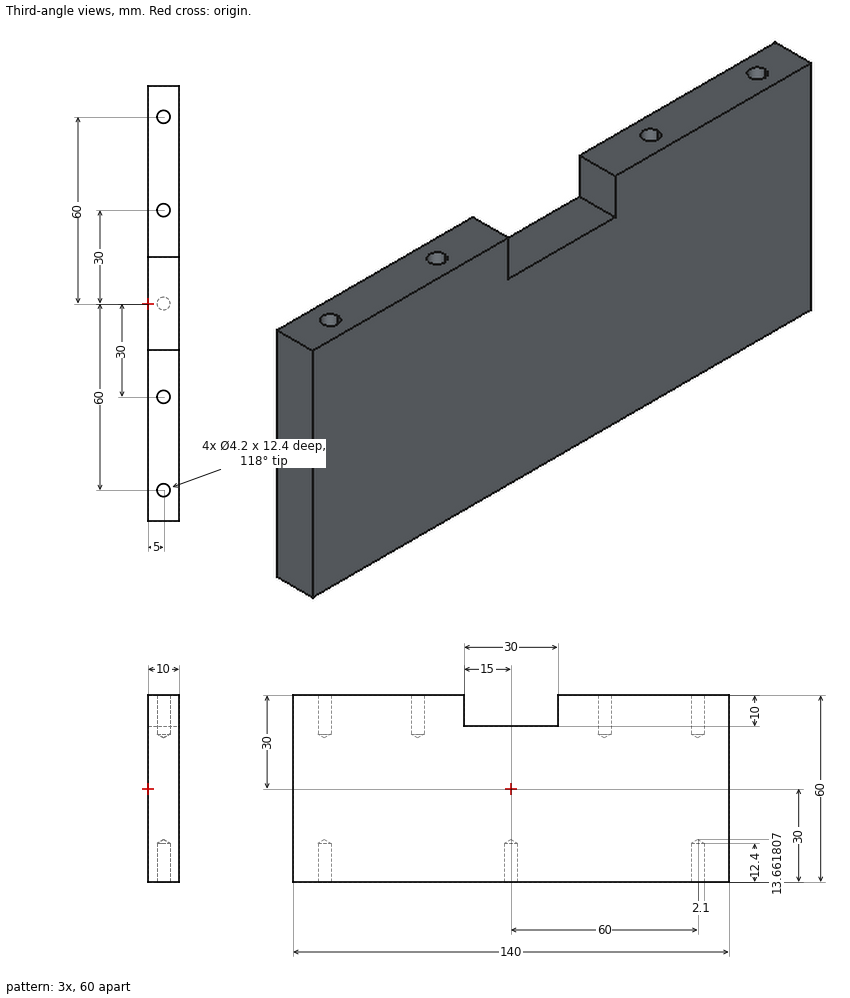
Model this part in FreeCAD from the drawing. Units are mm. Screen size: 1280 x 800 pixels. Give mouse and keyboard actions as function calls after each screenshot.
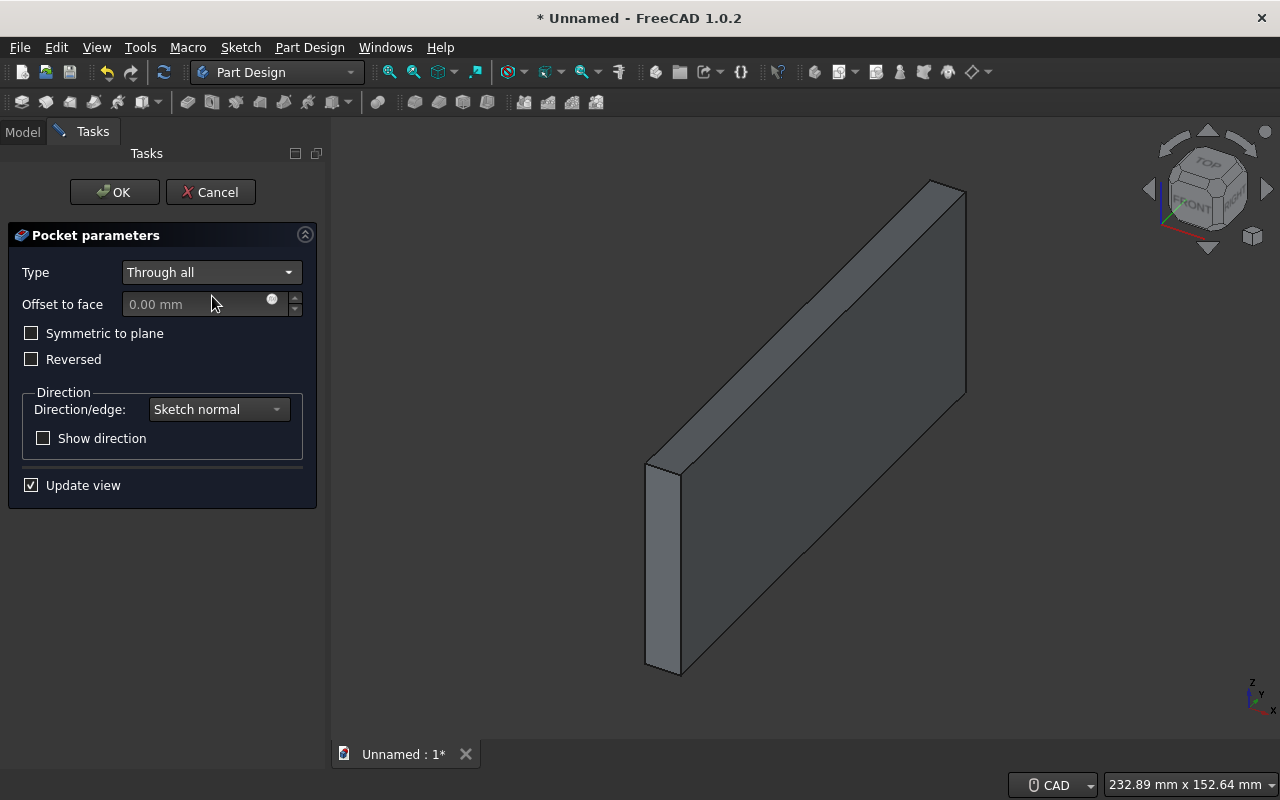
click(30, 359)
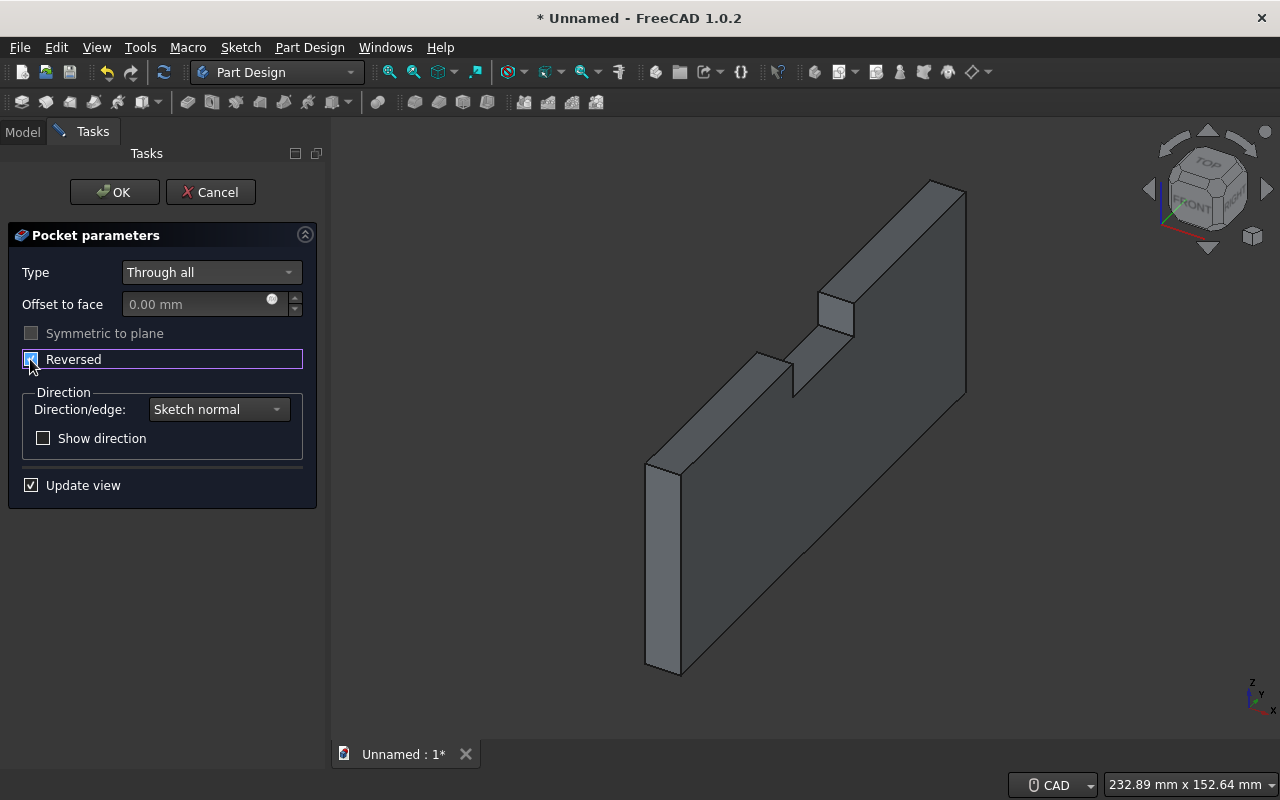
click(115, 192)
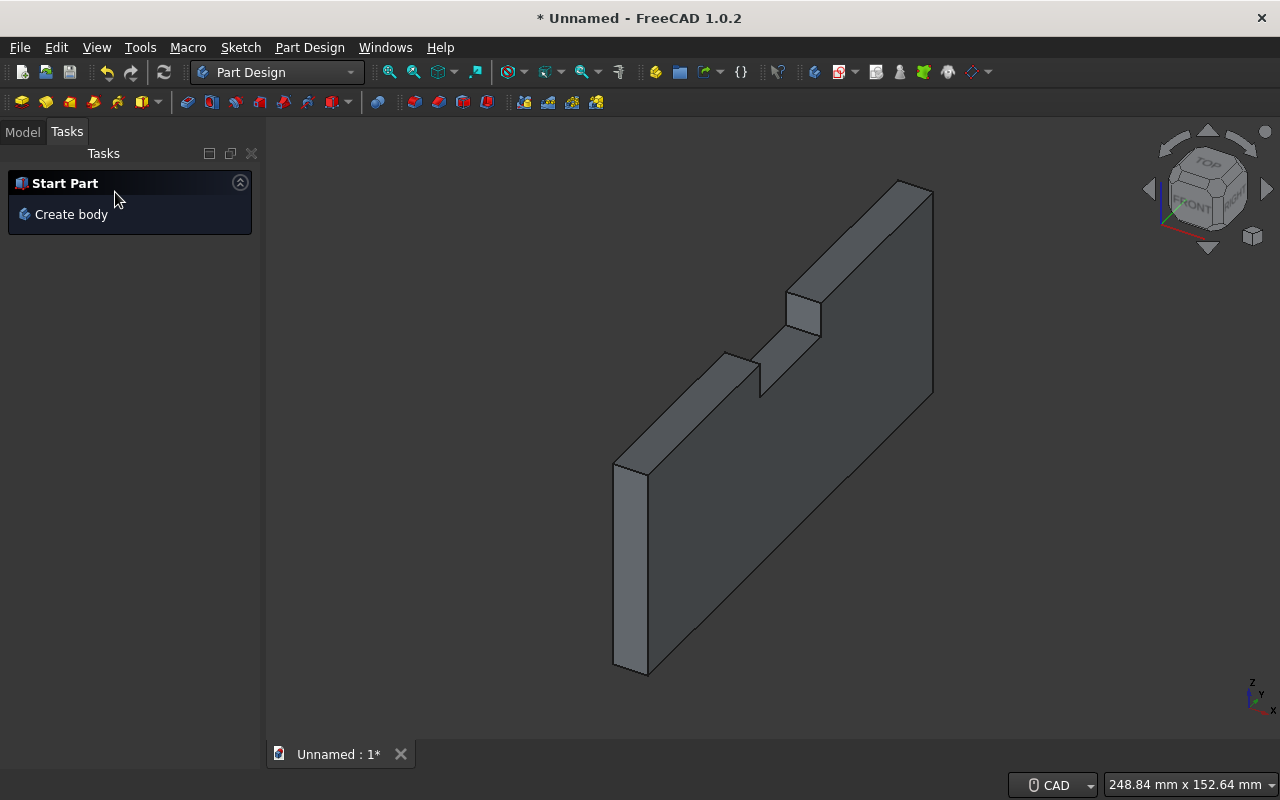
click(23, 131)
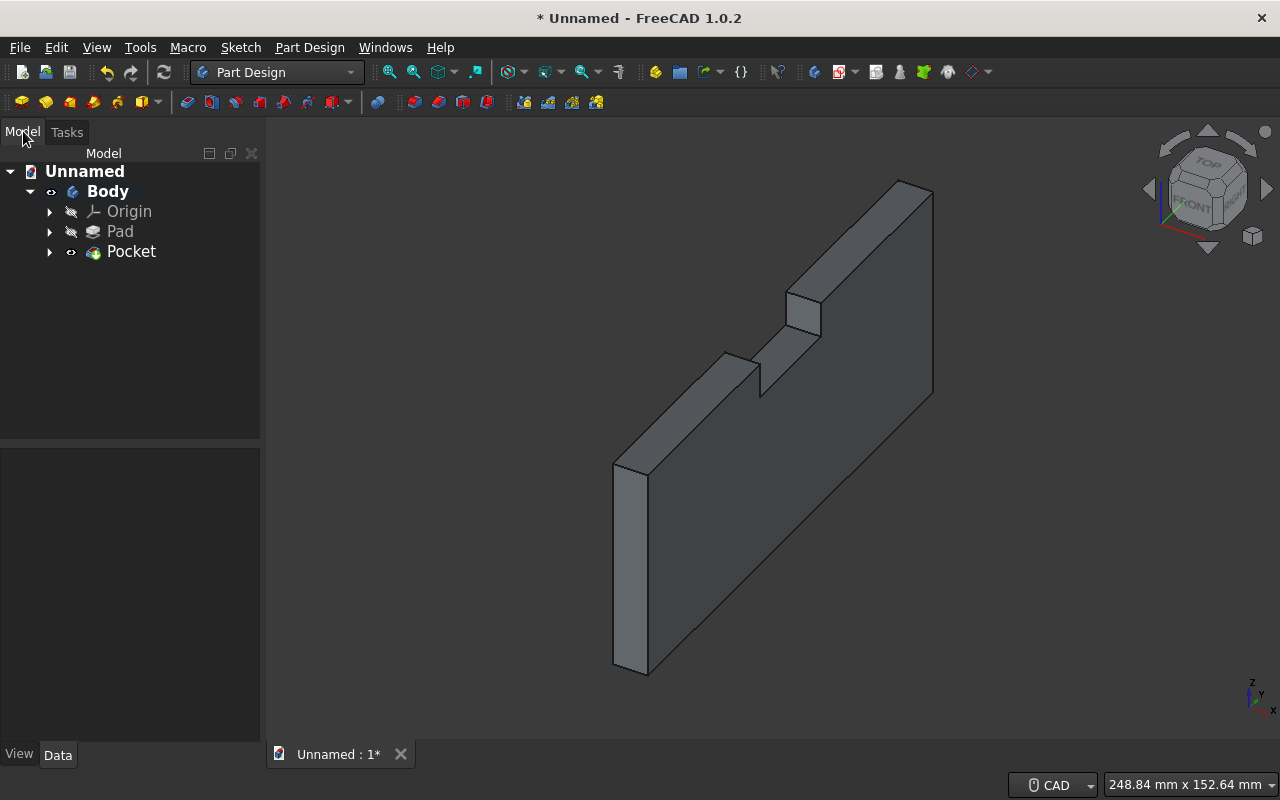
click(50, 212)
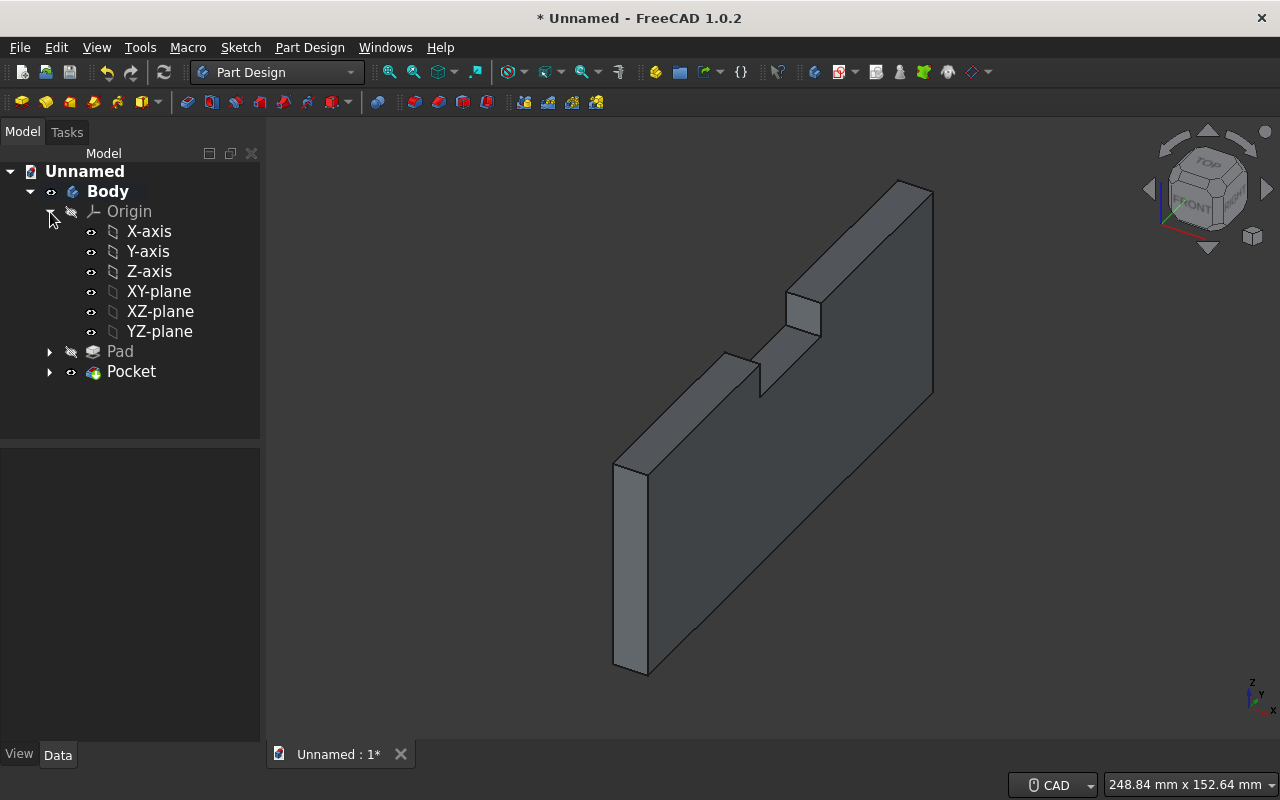
click(136, 332)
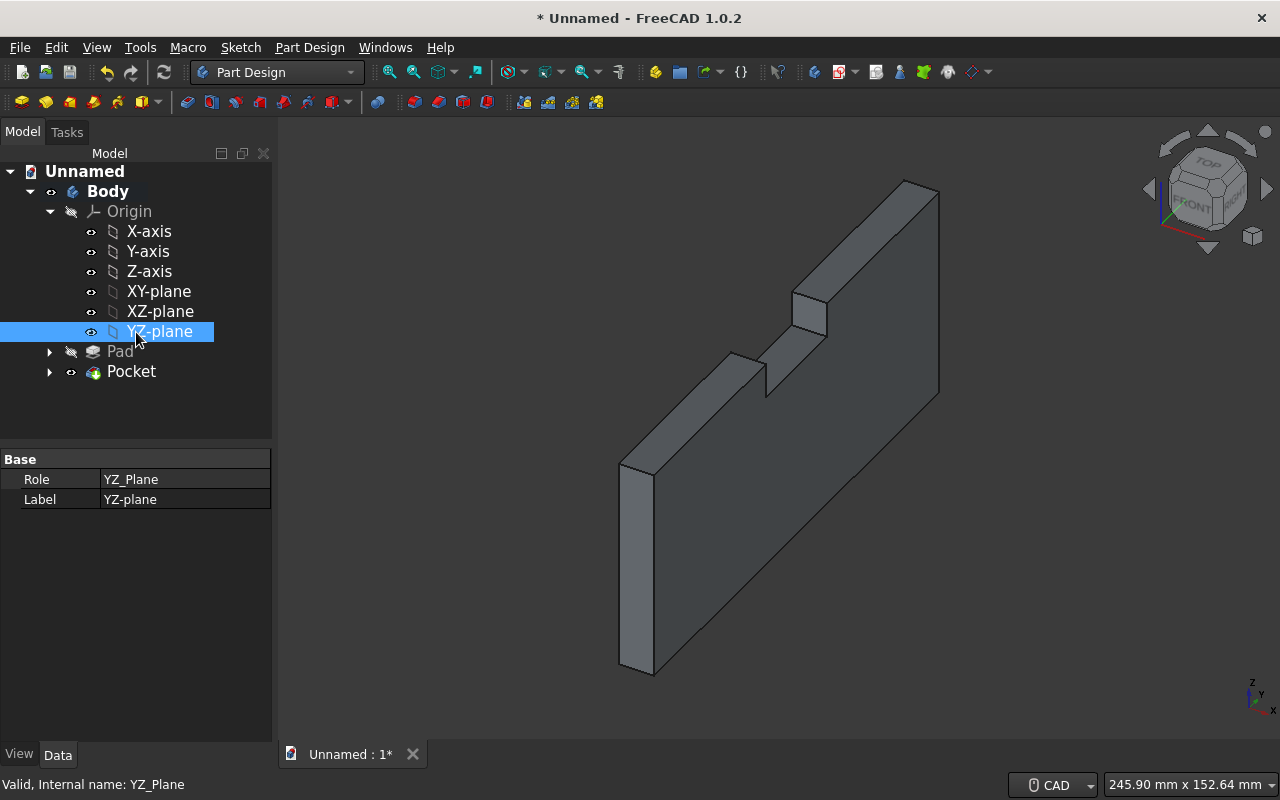
click(972, 72)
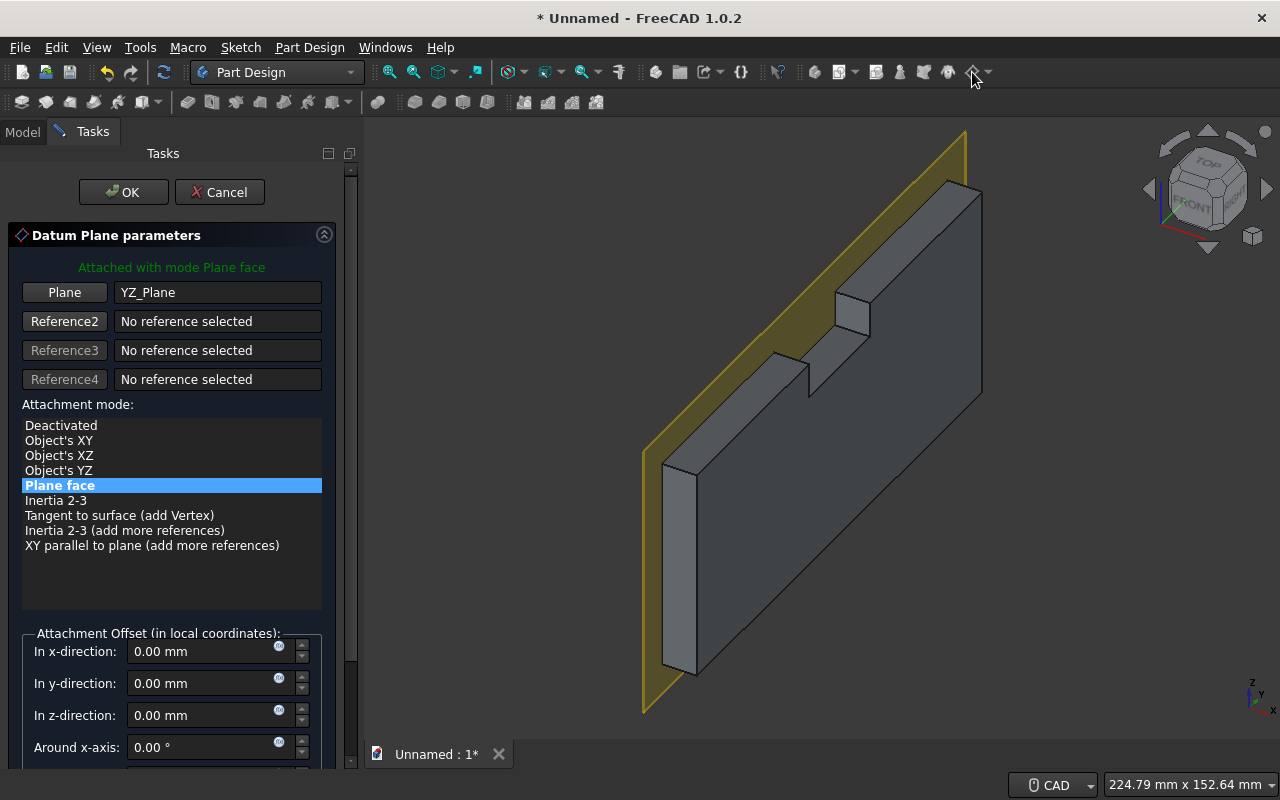
triple_click(210, 715)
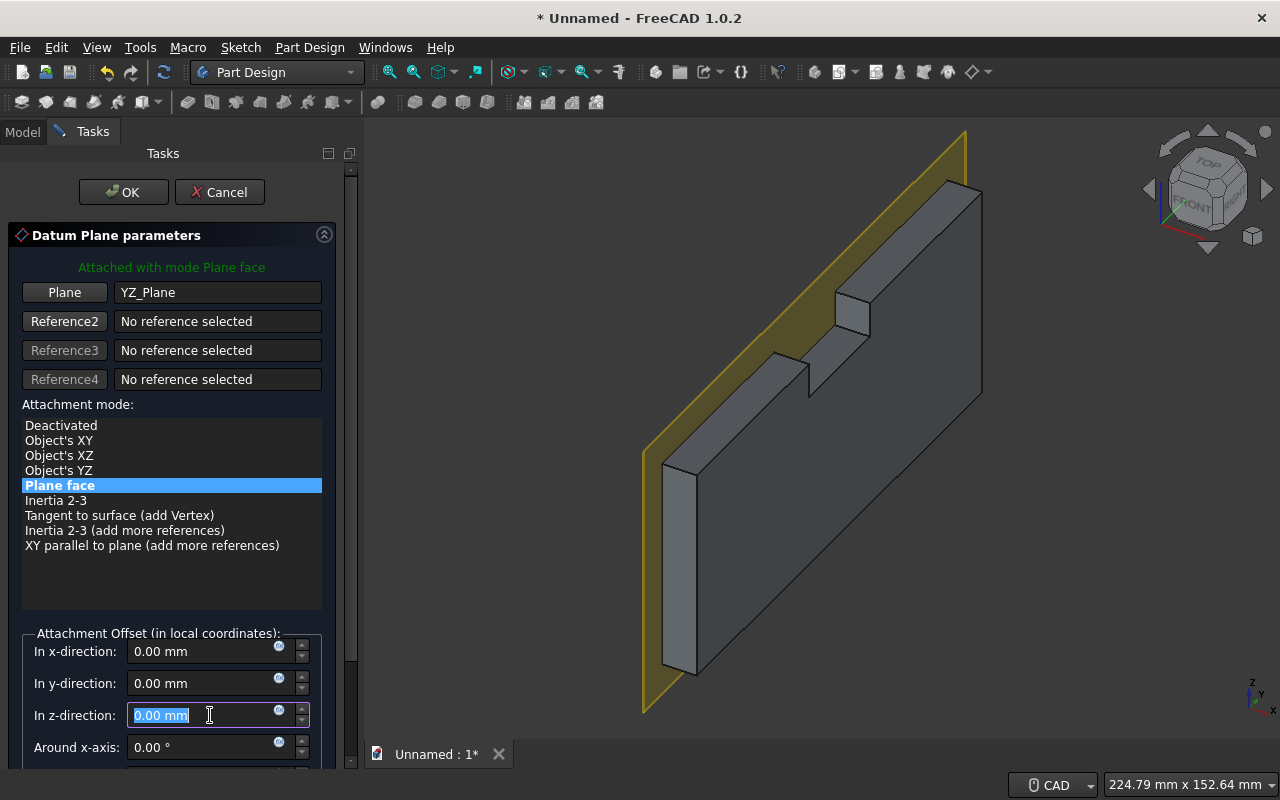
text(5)
key(Tab)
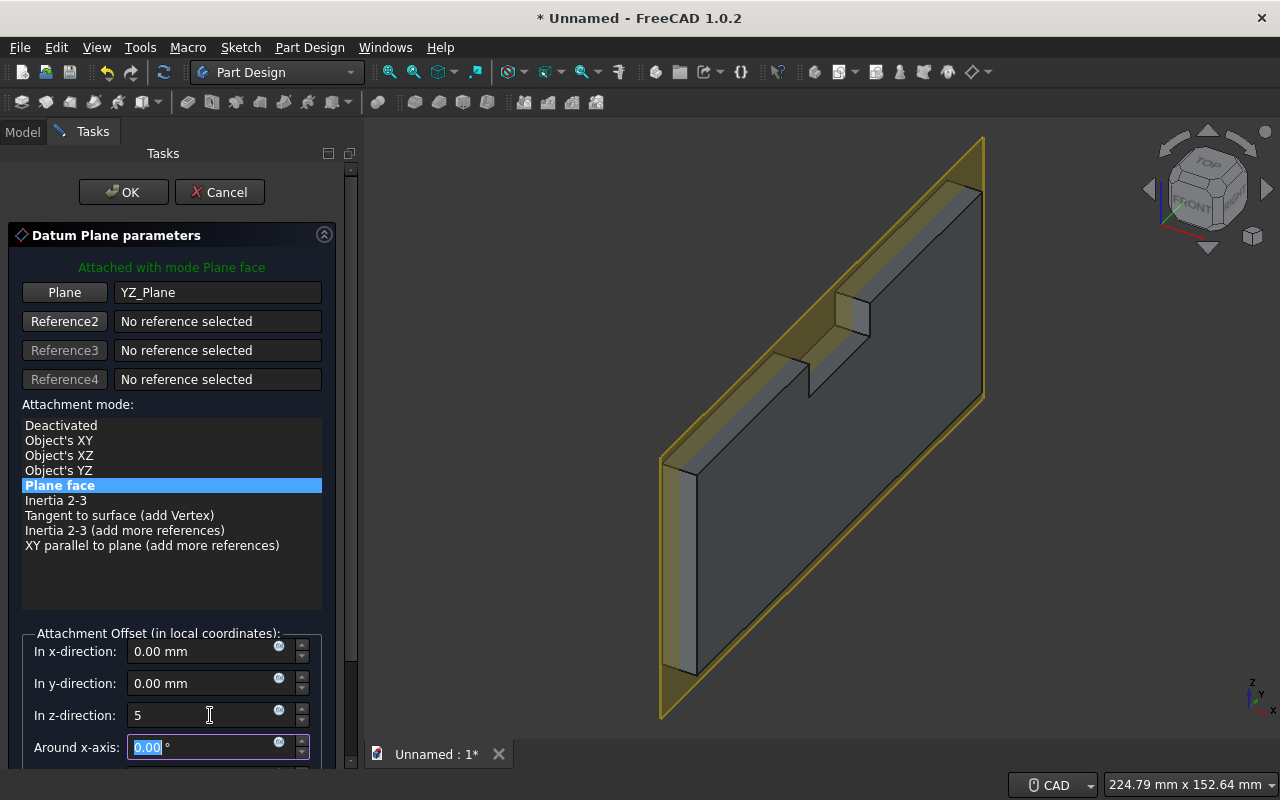
click(124, 192)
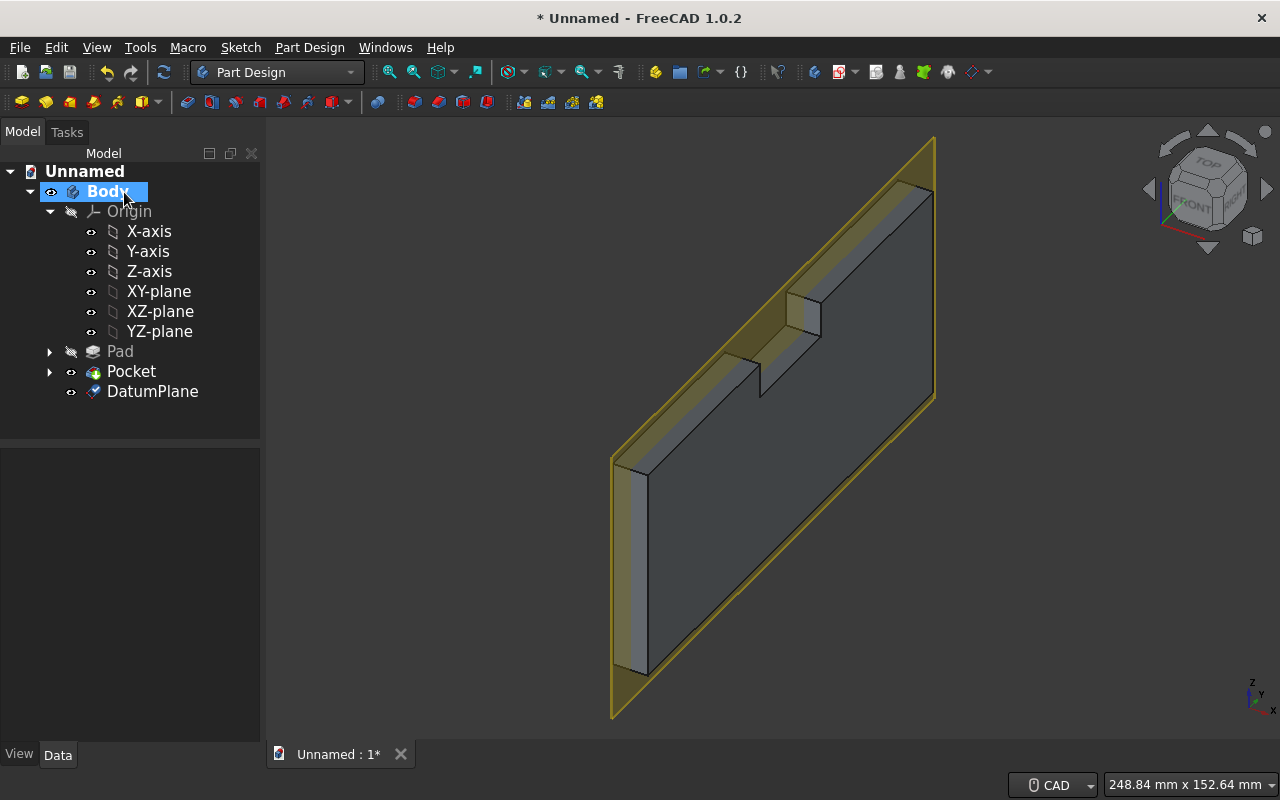
click(116, 392)